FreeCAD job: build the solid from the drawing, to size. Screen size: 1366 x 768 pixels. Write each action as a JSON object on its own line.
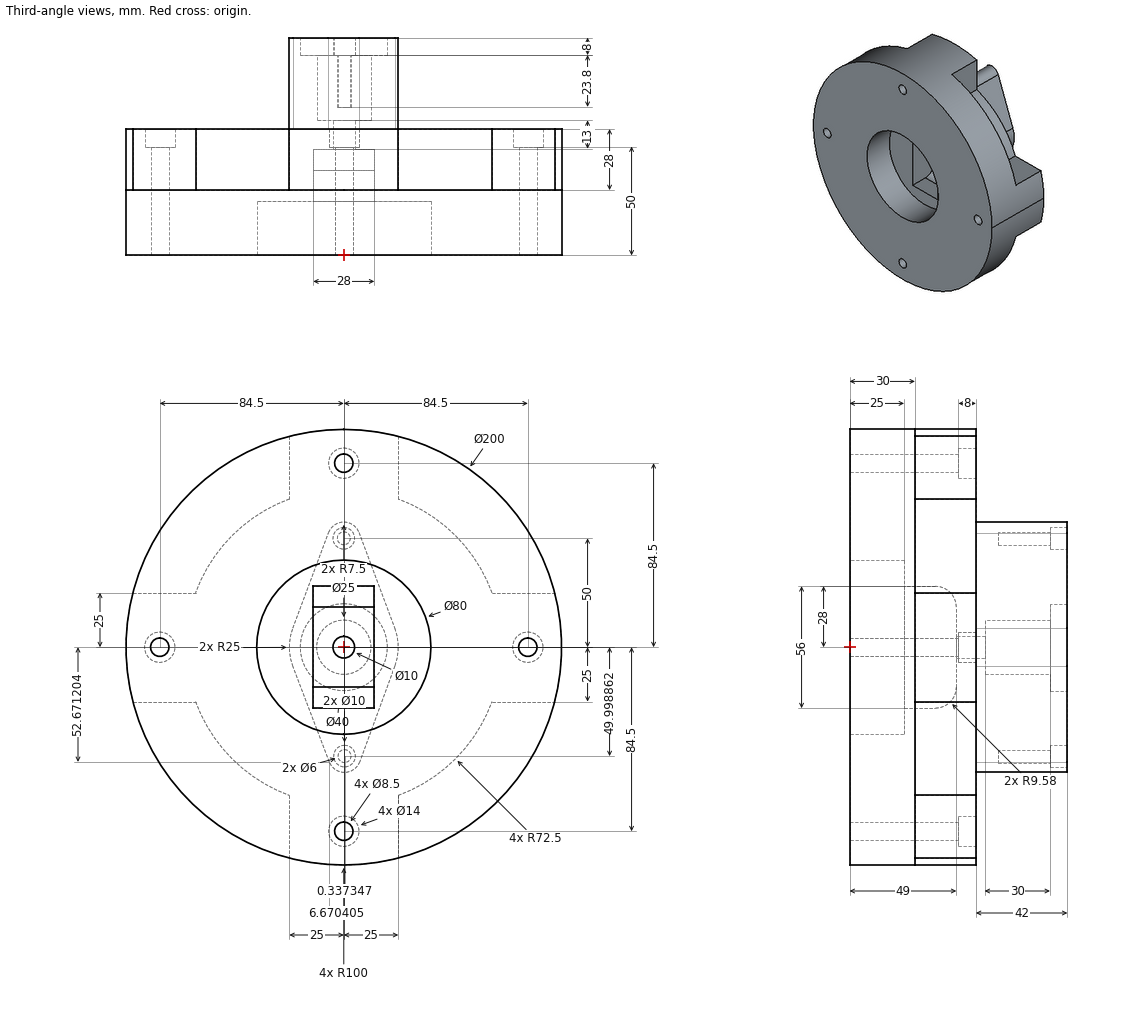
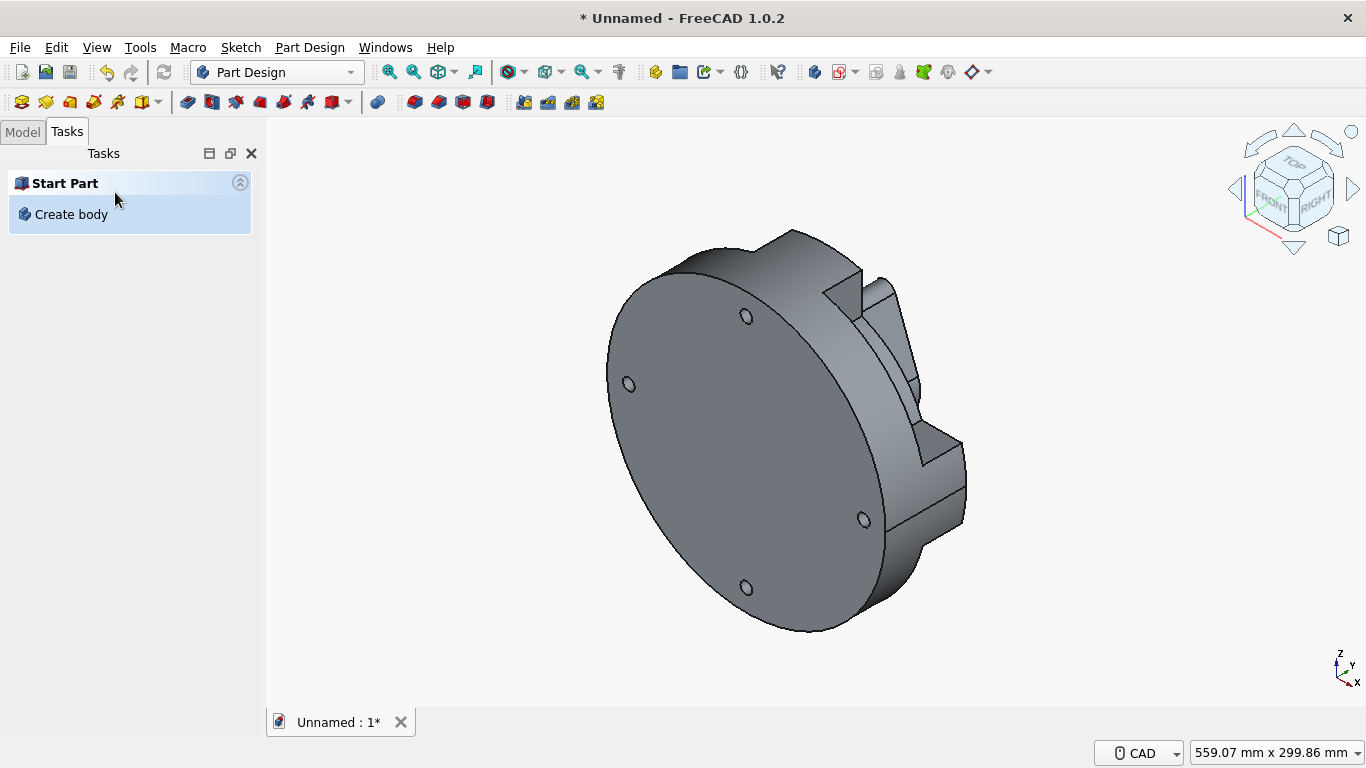
{"action": "left_click", "coordinate": [746, 451]}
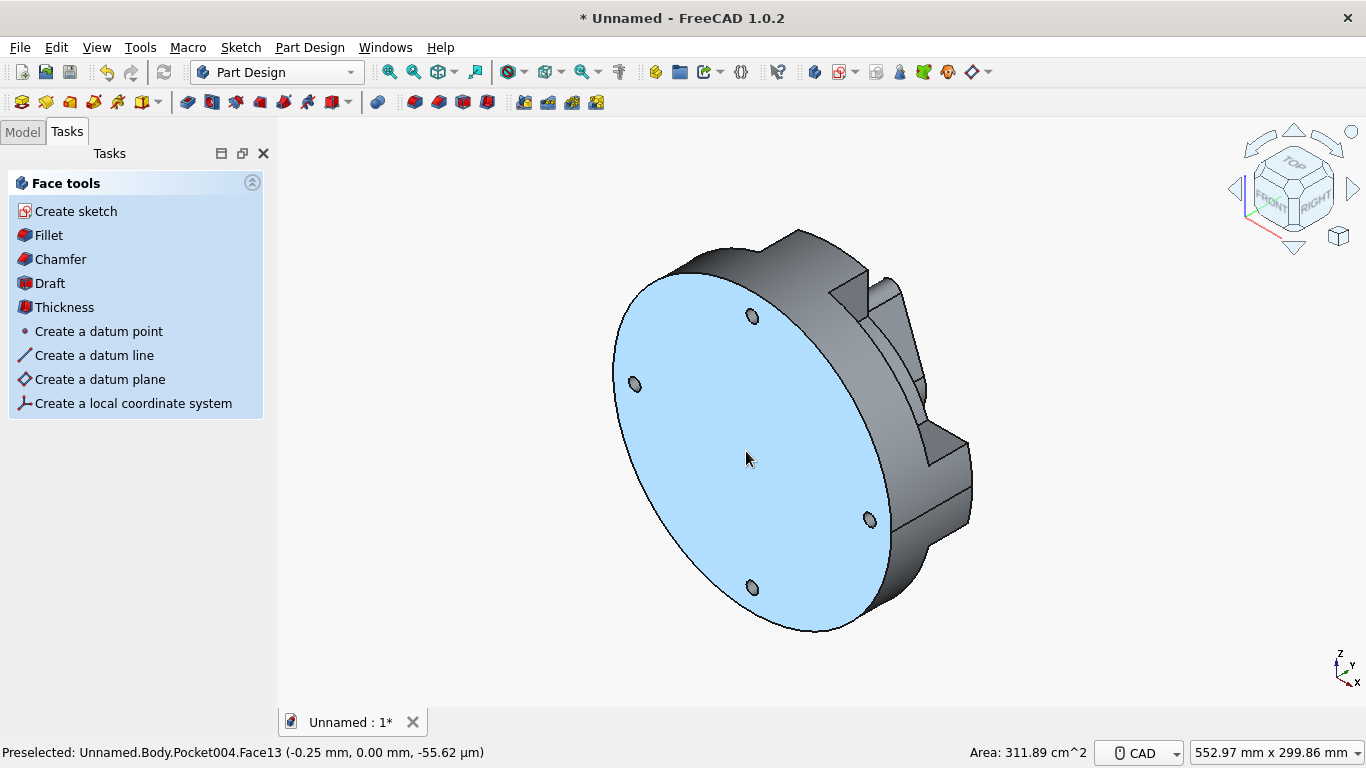
{"action": "left_click", "coordinate": [840, 72]}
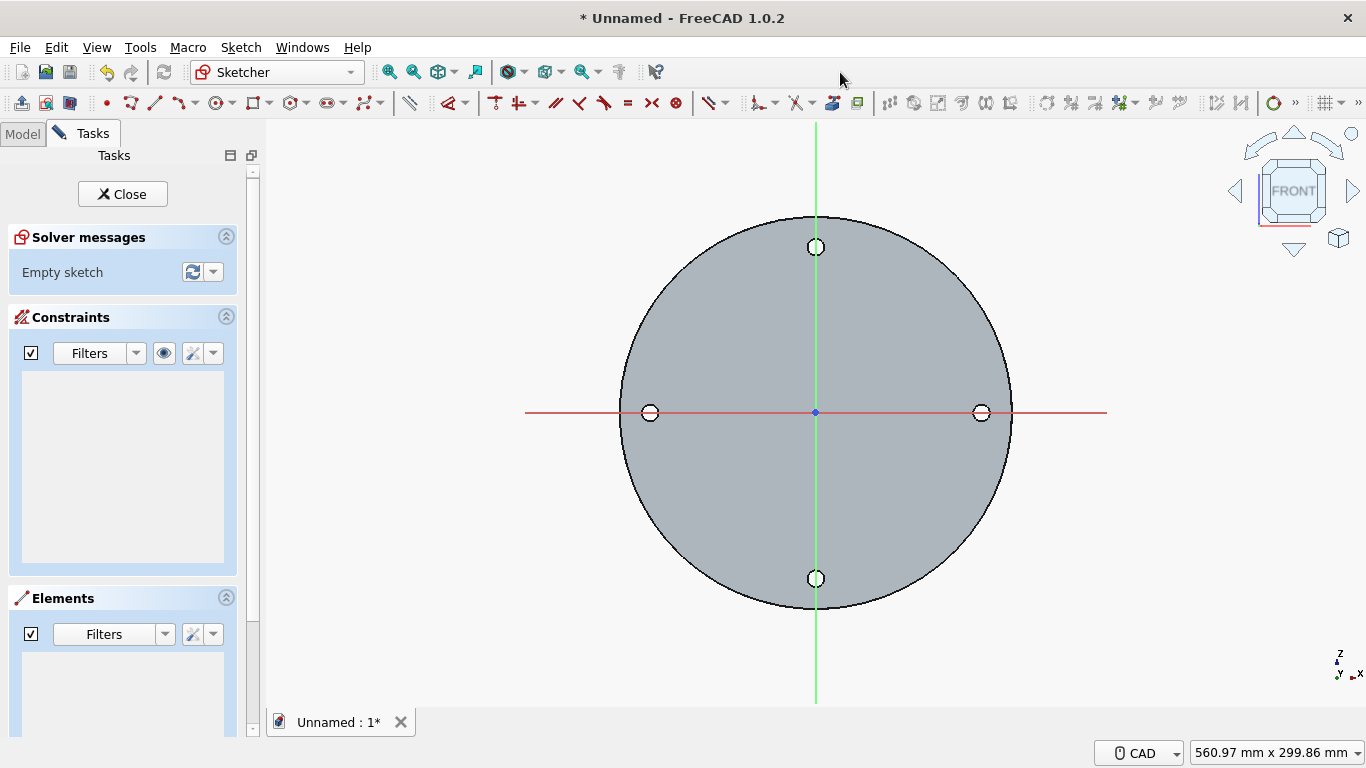
{"action": "scroll", "coordinate": [872, 413], "scroll_direction": "up", "scroll_amount": 4}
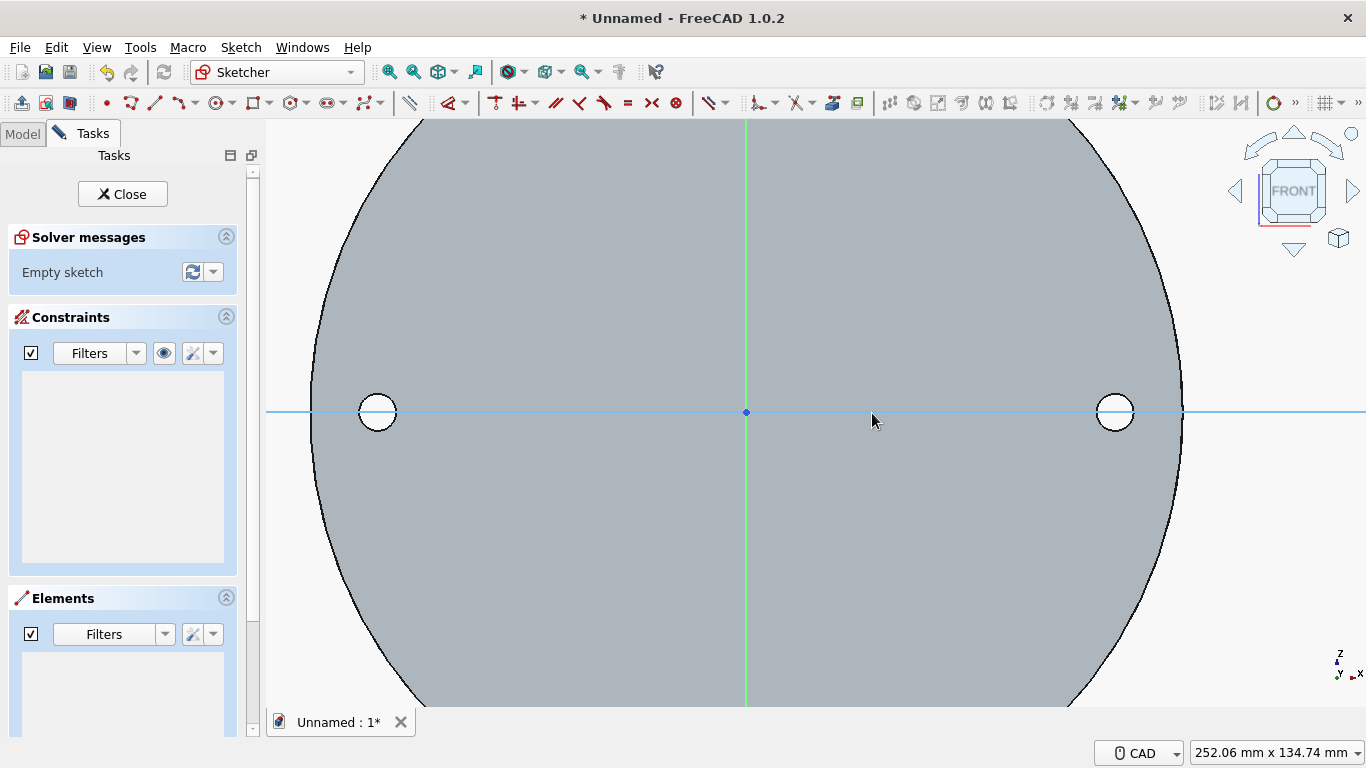
{"action": "key", "text": "g c"}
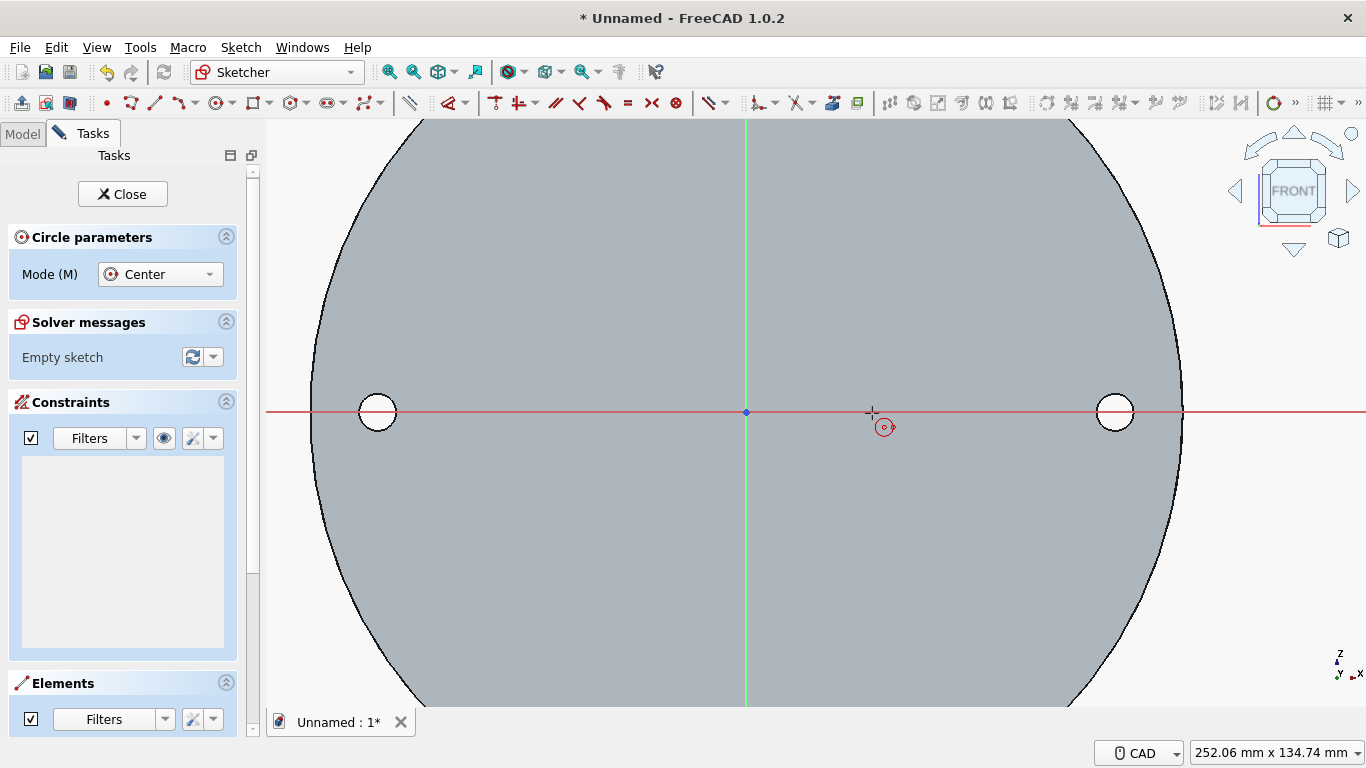
{"action": "left_click", "coordinate": [746, 412]}
{"action": "left_click", "coordinate": [870, 289]}
{"action": "key", "text": "Escape"}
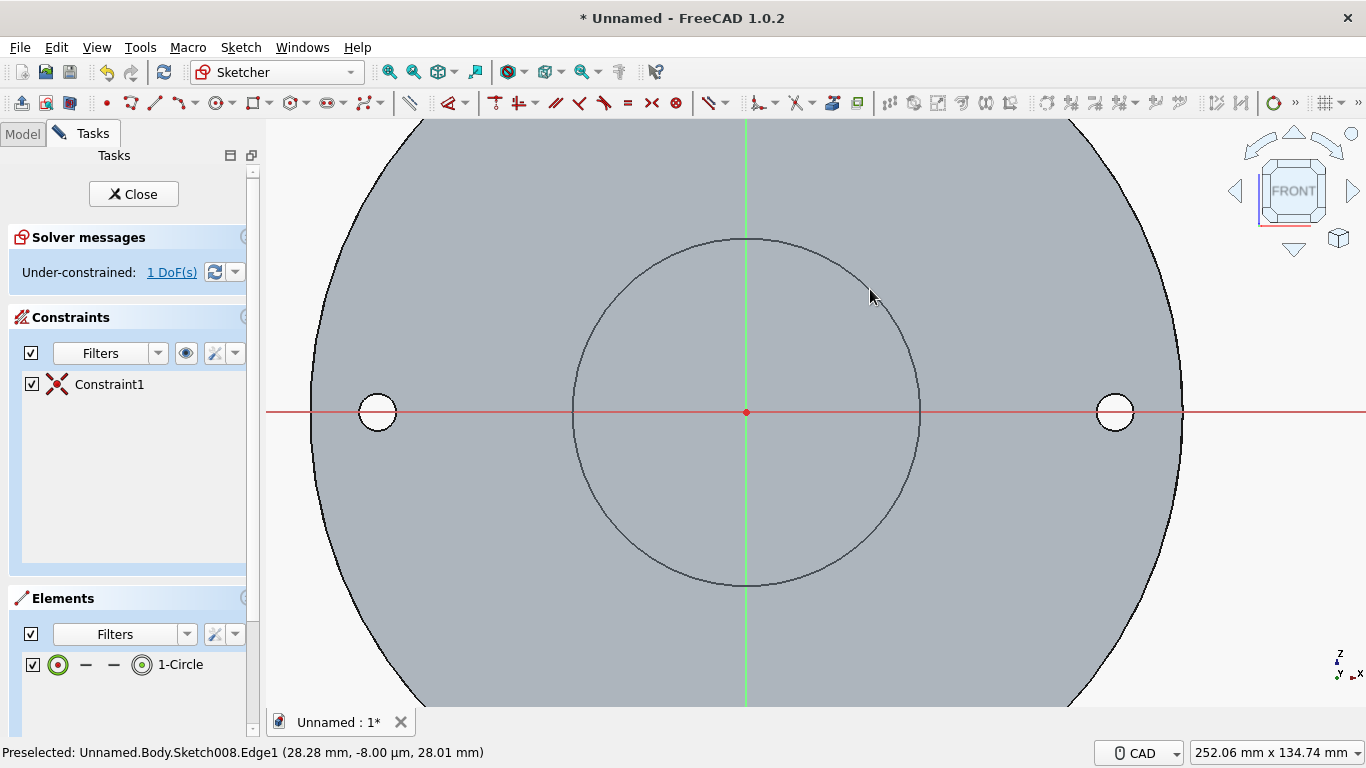
{"action": "key", "text": "d"}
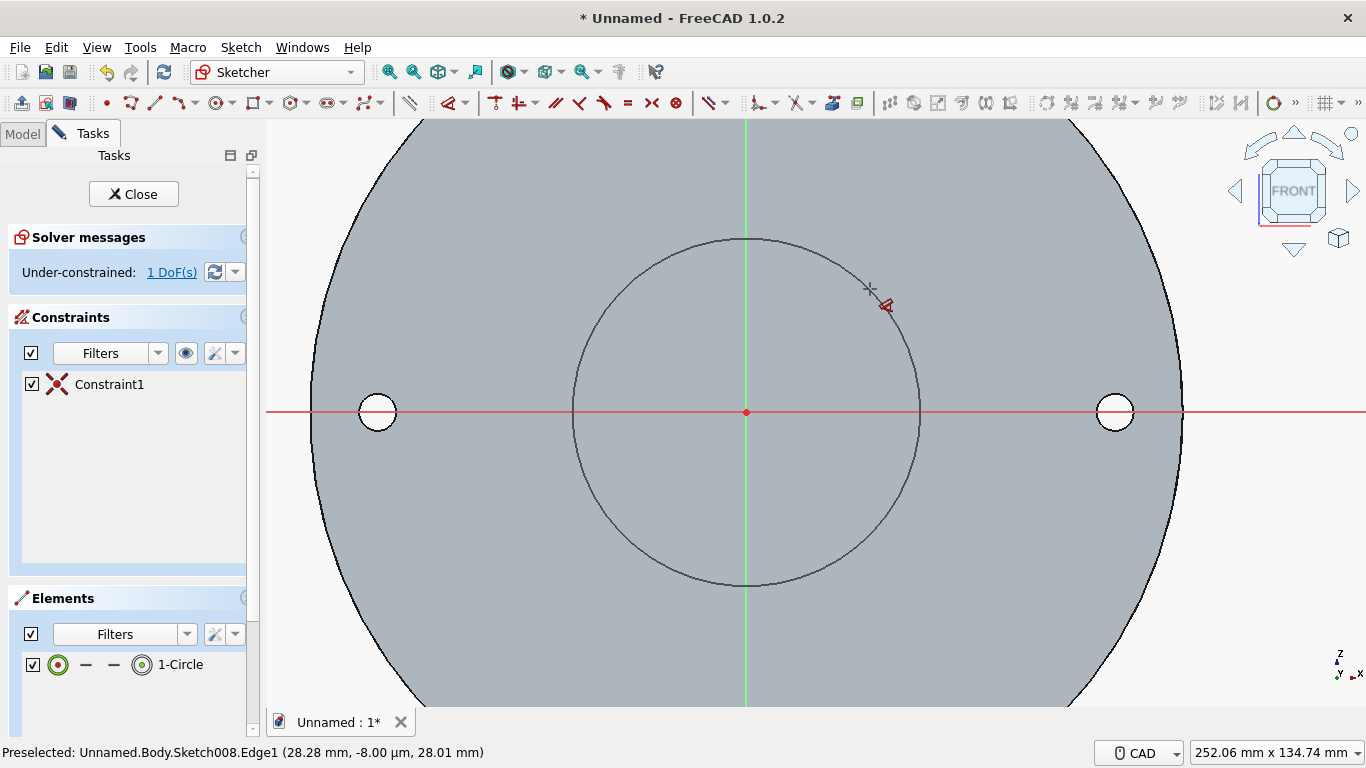
{"action": "left_click", "coordinate": [869, 289]}
{"action": "left_click", "coordinate": [892, 266]}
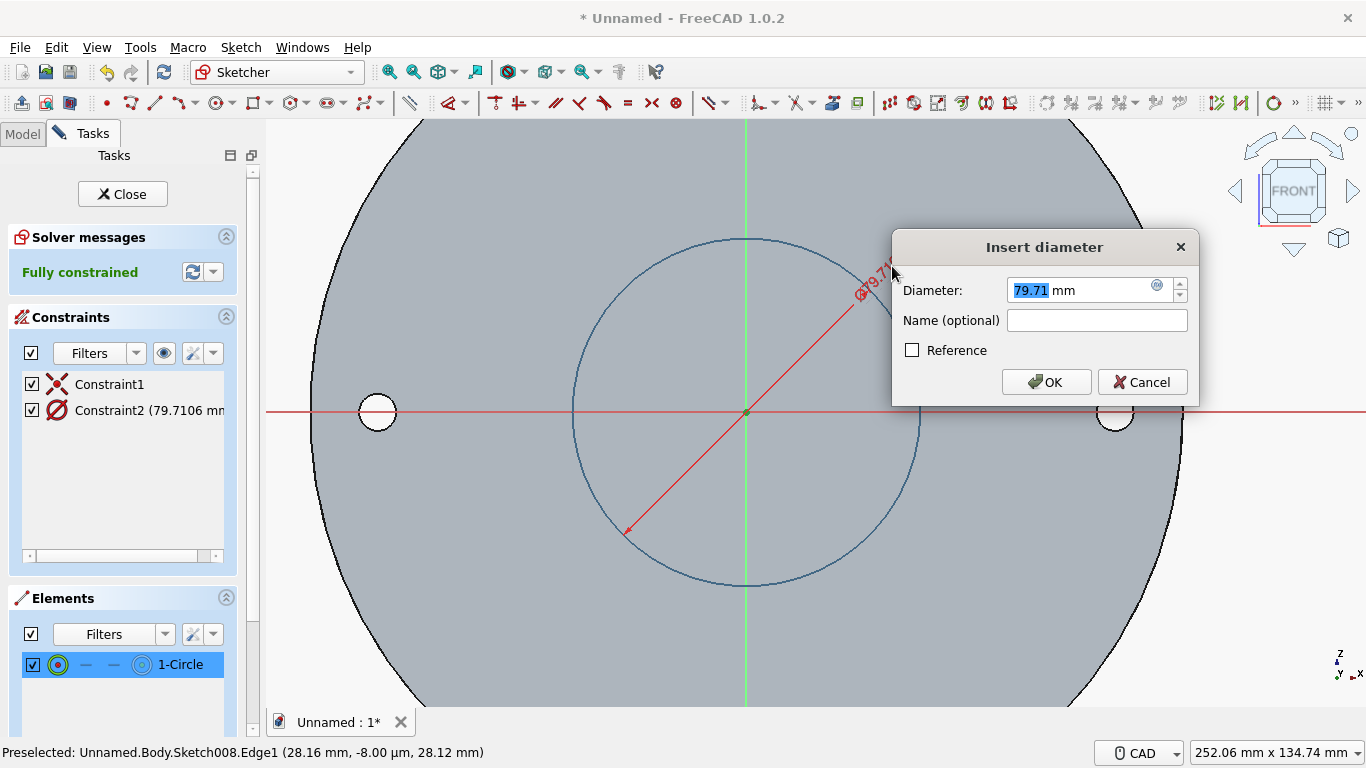
{"action": "type", "text": "80"}
{"action": "key", "text": "Return"}
{"action": "key", "text": "Escape"}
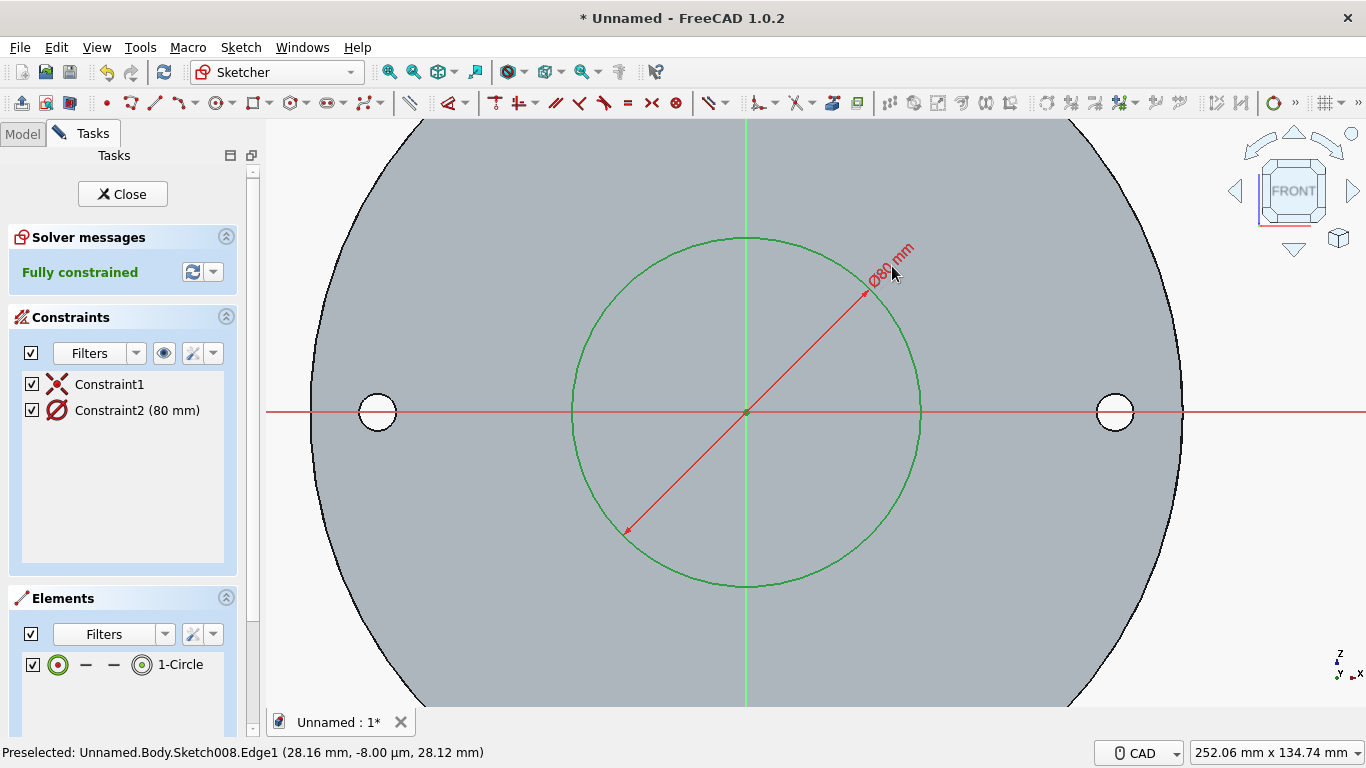
{"action": "left_click", "coordinate": [123, 194]}